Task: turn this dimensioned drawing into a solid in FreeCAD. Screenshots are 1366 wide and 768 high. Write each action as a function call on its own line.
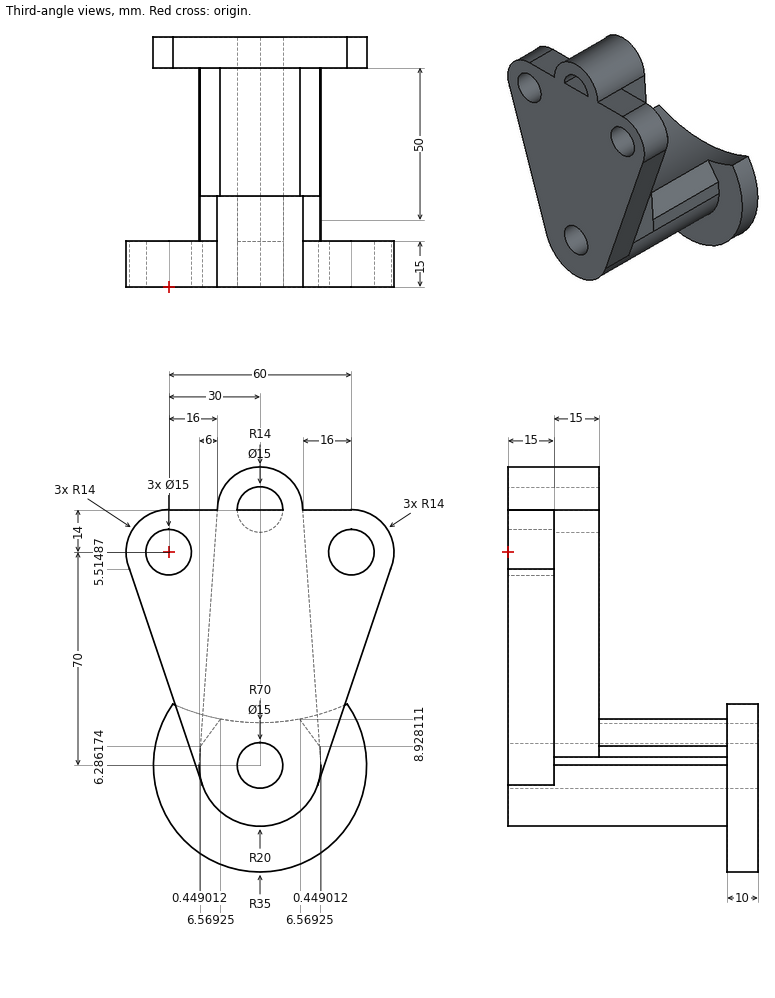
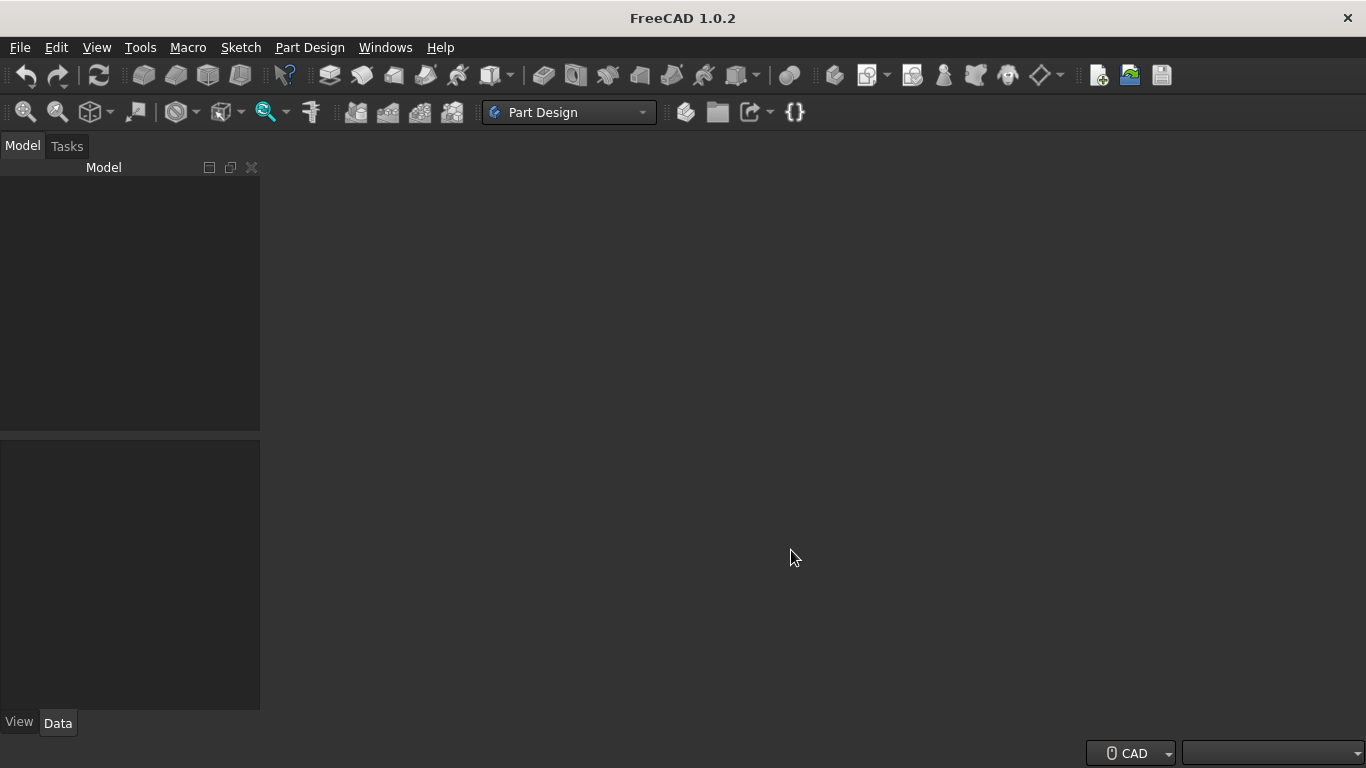
click(1098, 76)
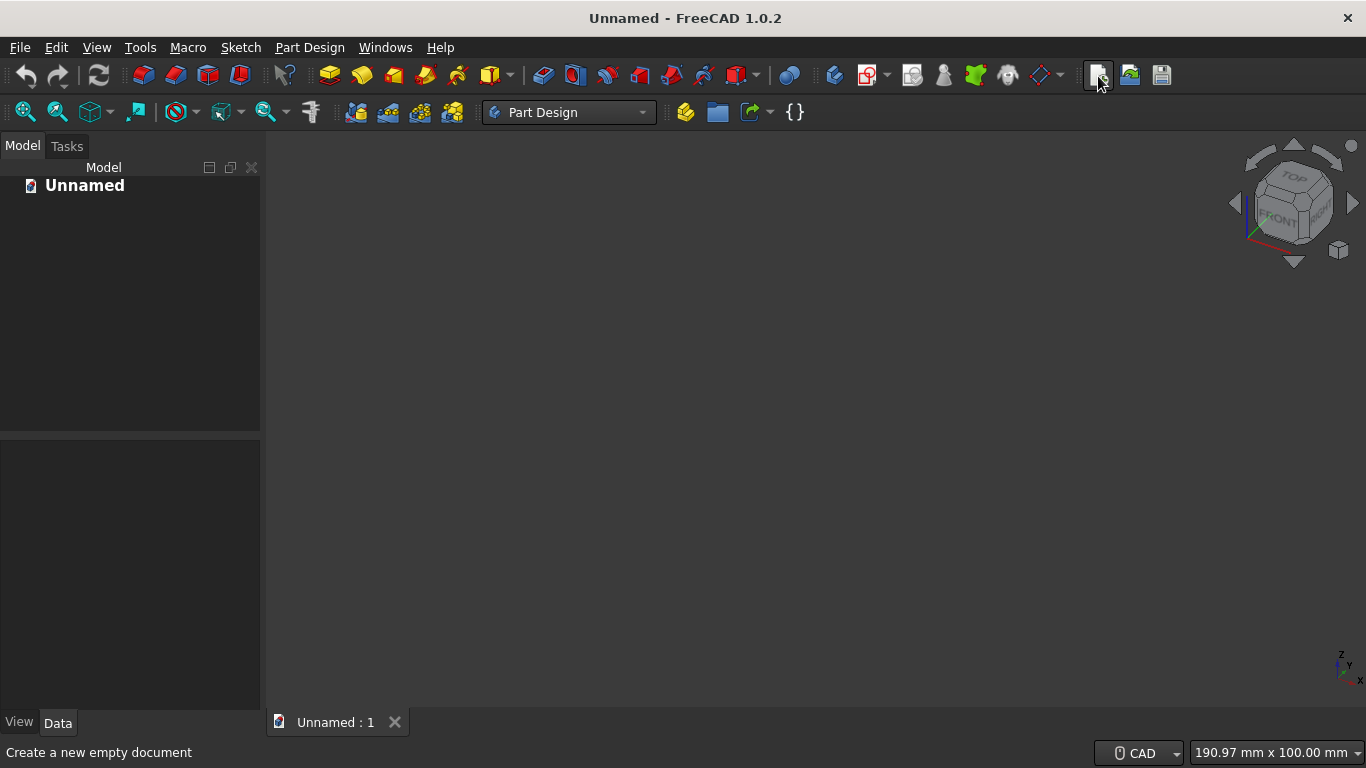
click(868, 76)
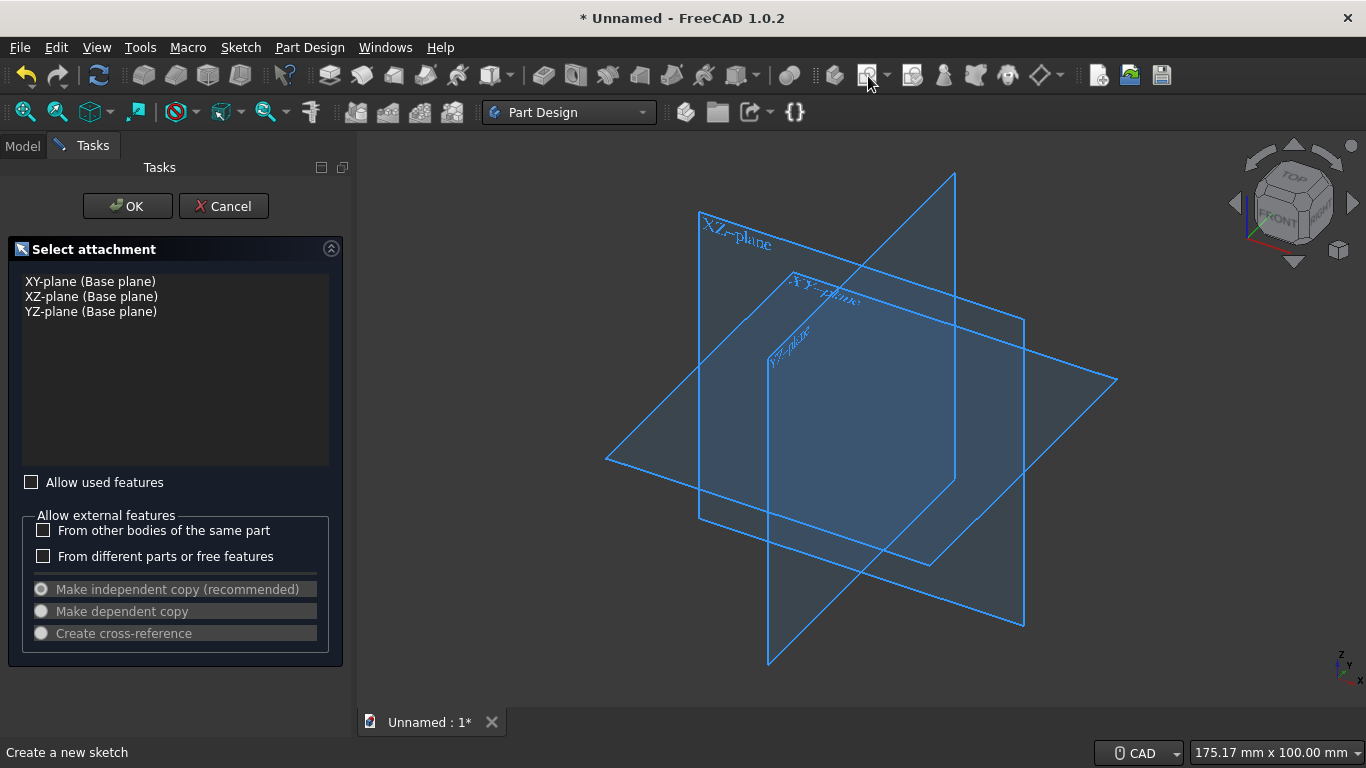
click(82, 296)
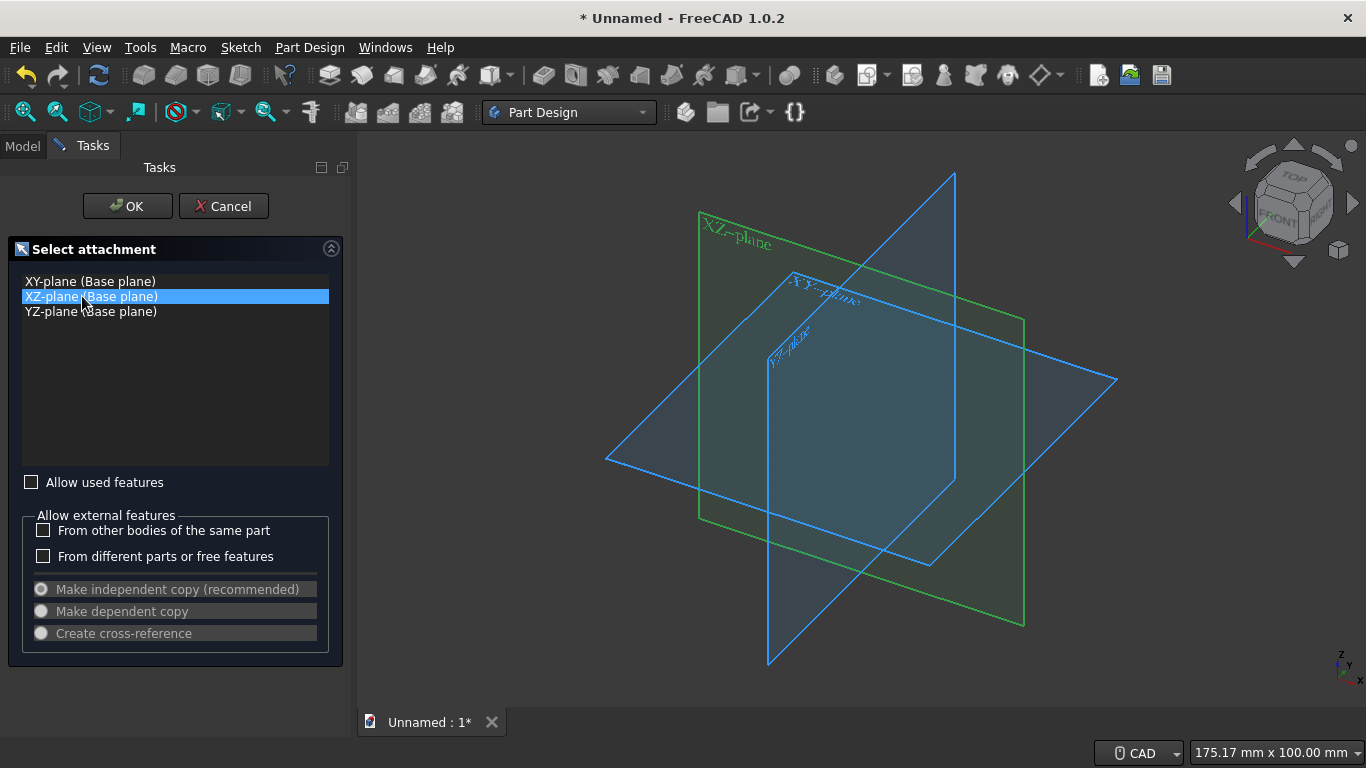
click(128, 206)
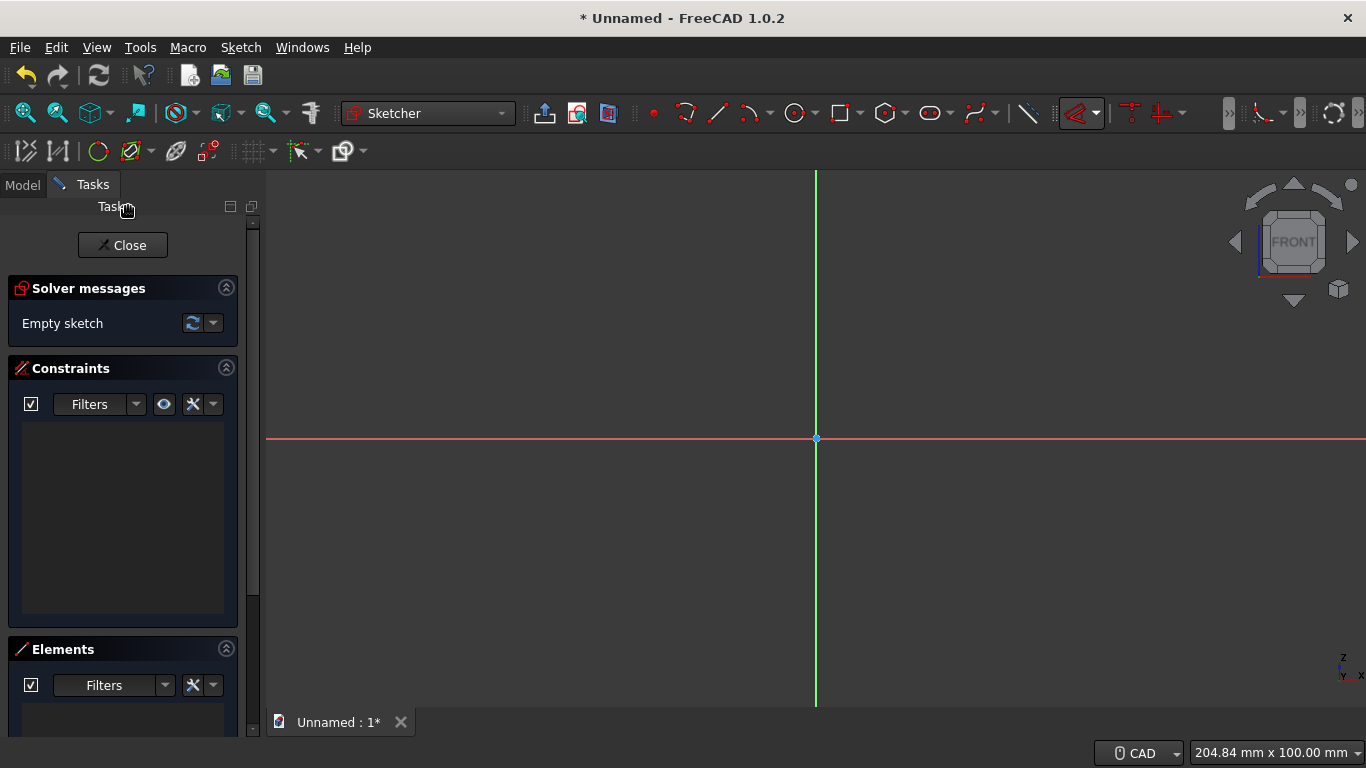
scroll(468, 210, down, 3)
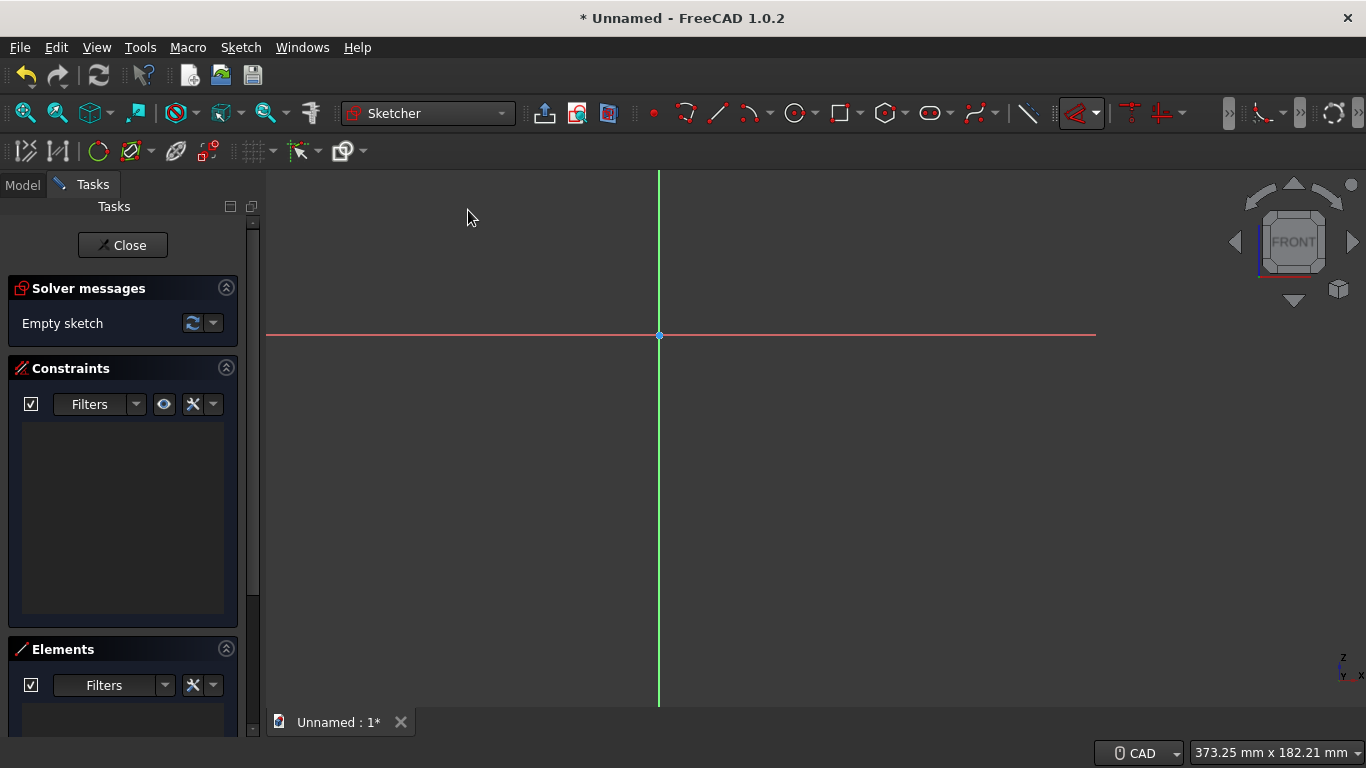
click(718, 114)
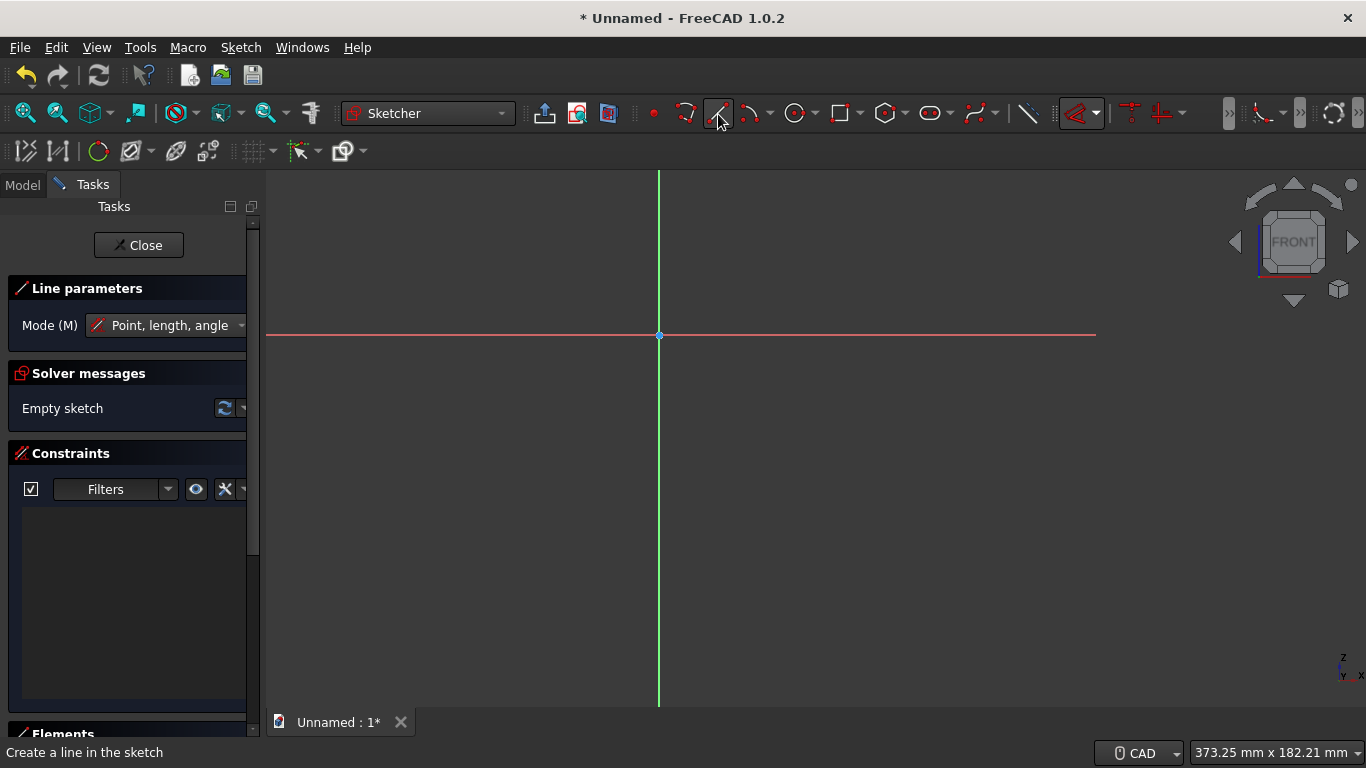
click(710, 558)
click(621, 352)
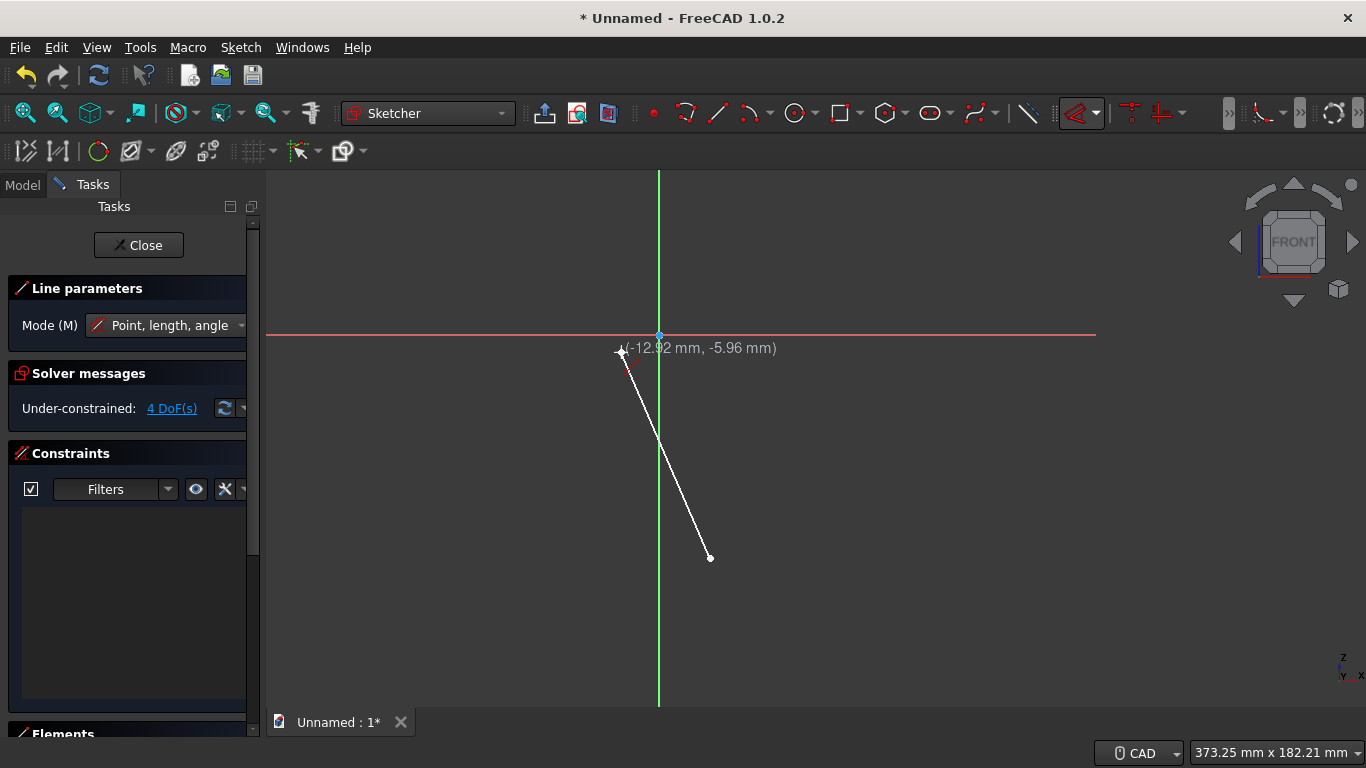
click(659, 294)
click(836, 294)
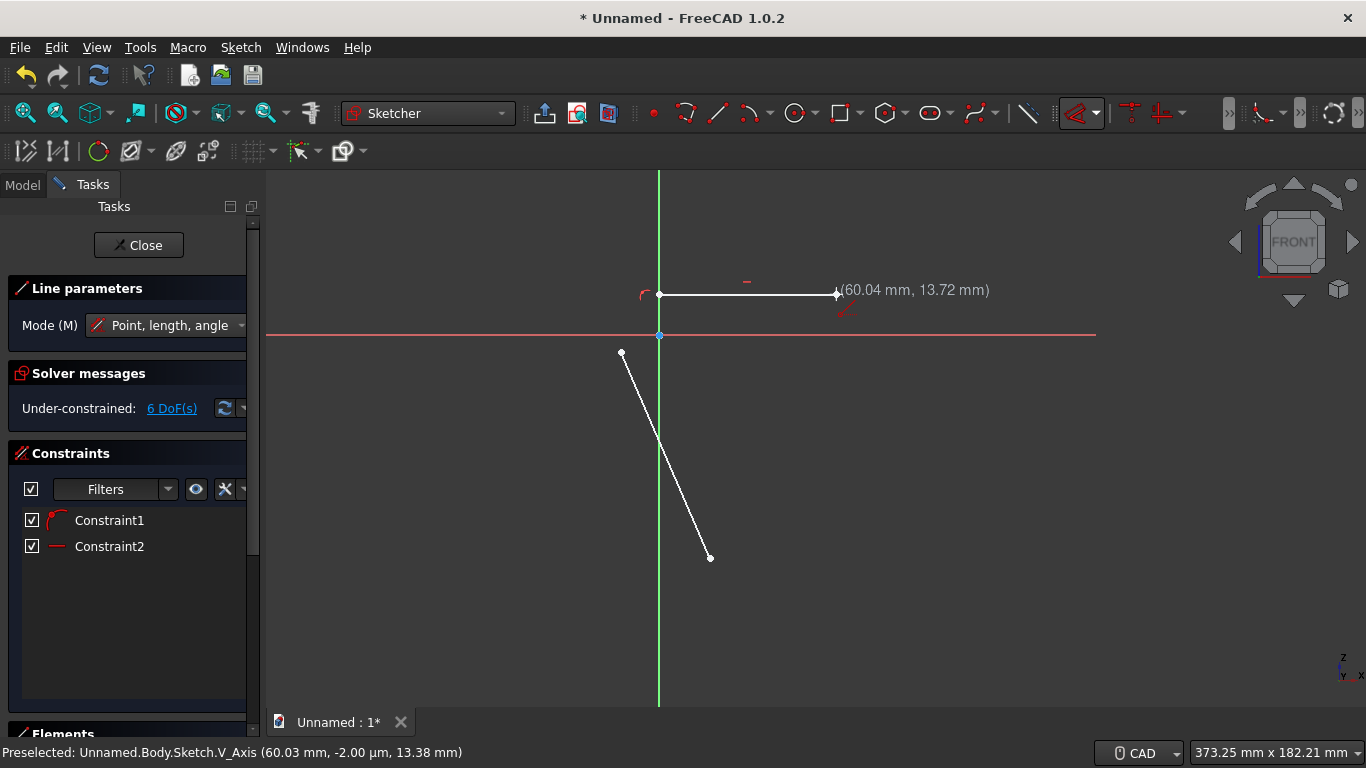
click(874, 352)
click(785, 558)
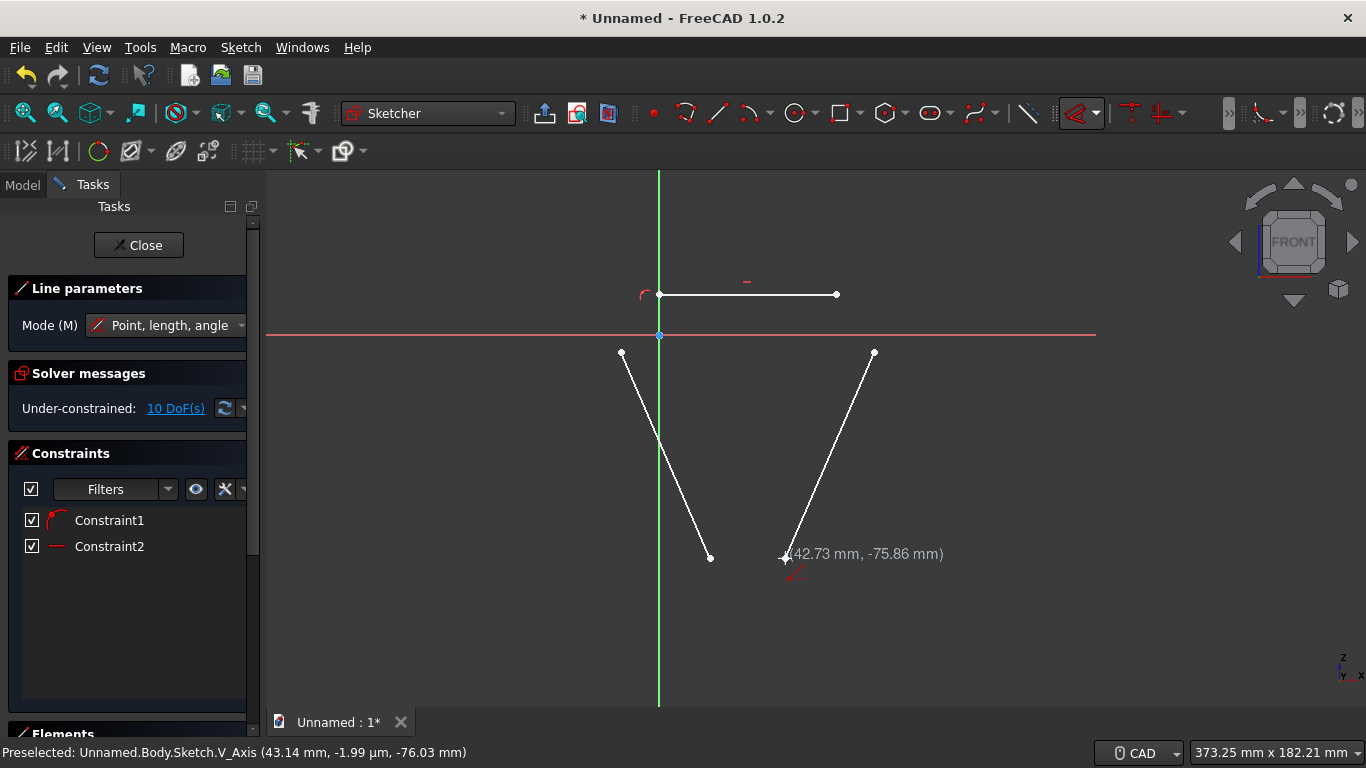
click(772, 114)